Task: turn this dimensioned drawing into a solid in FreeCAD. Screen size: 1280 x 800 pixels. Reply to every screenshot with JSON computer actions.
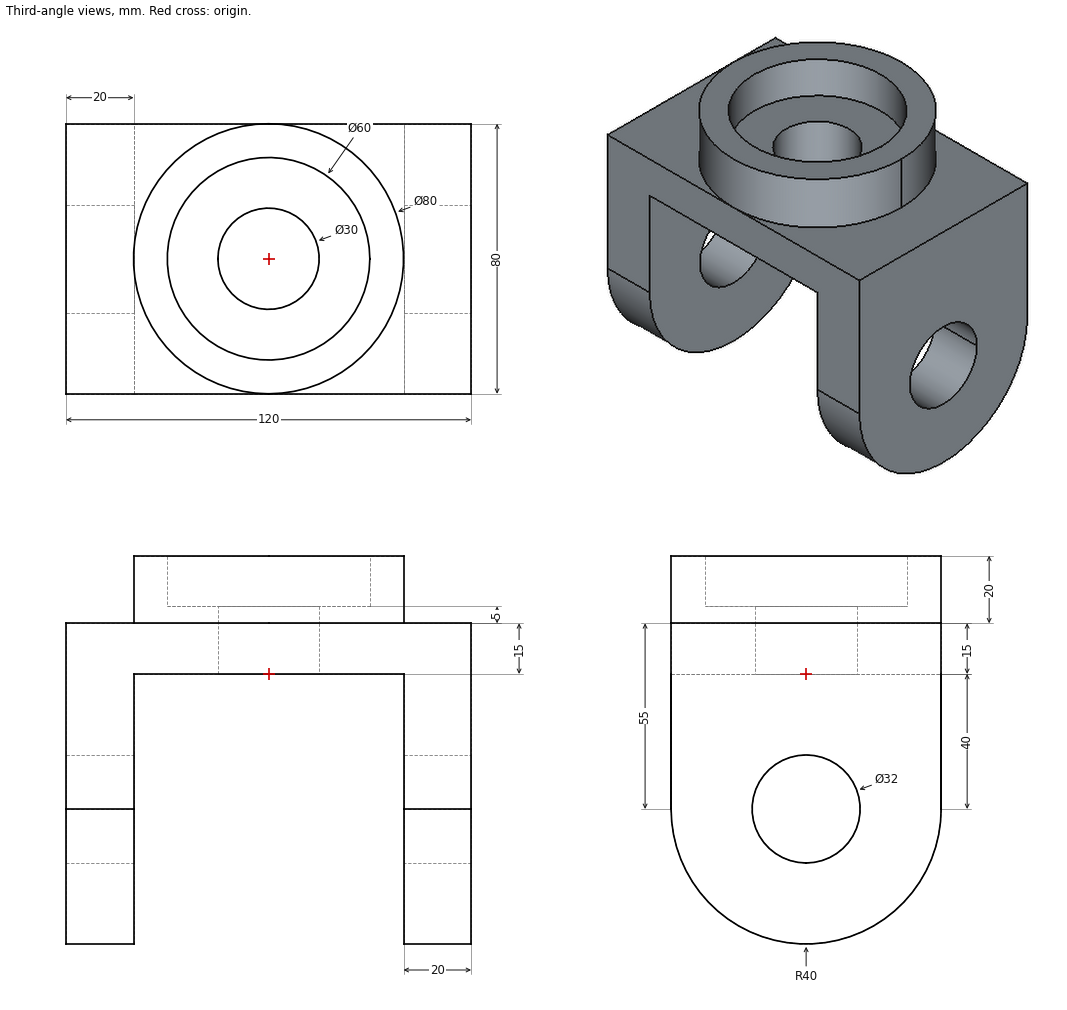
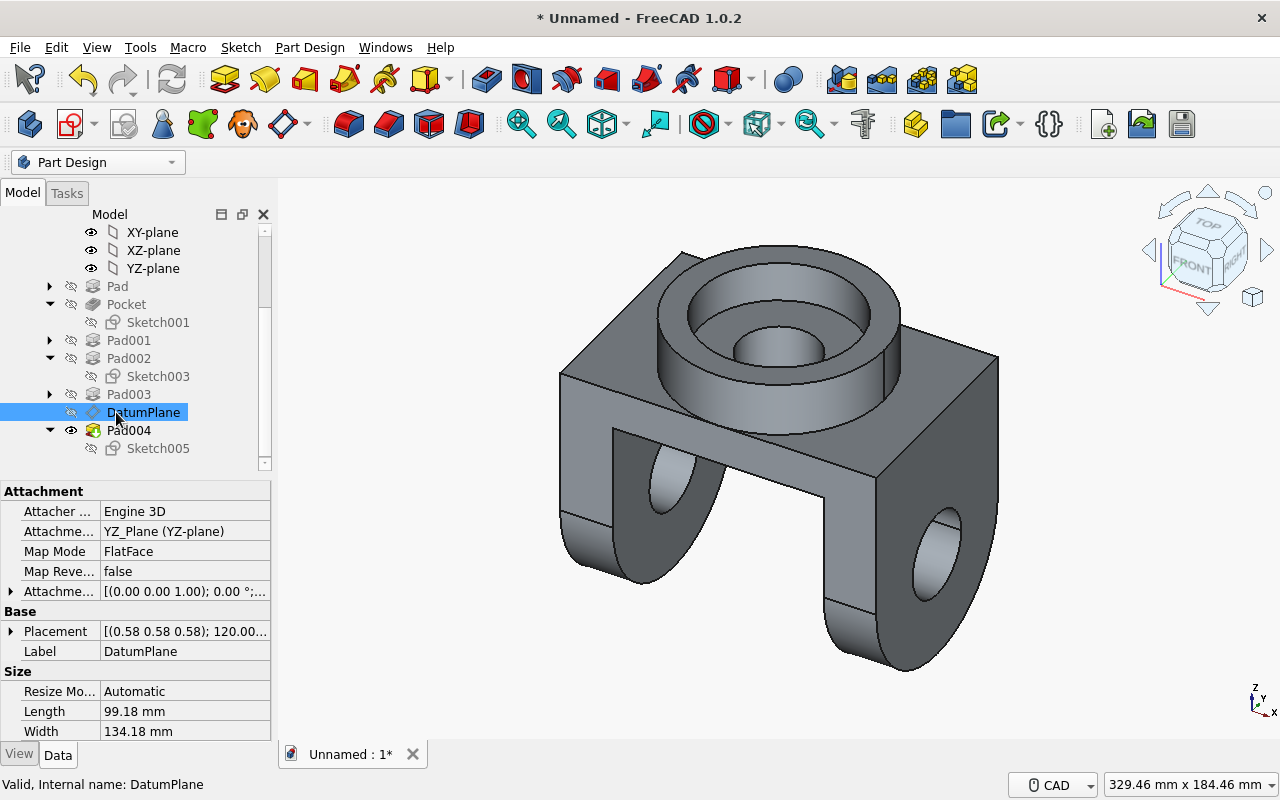
{"action": "key", "text": "0"}